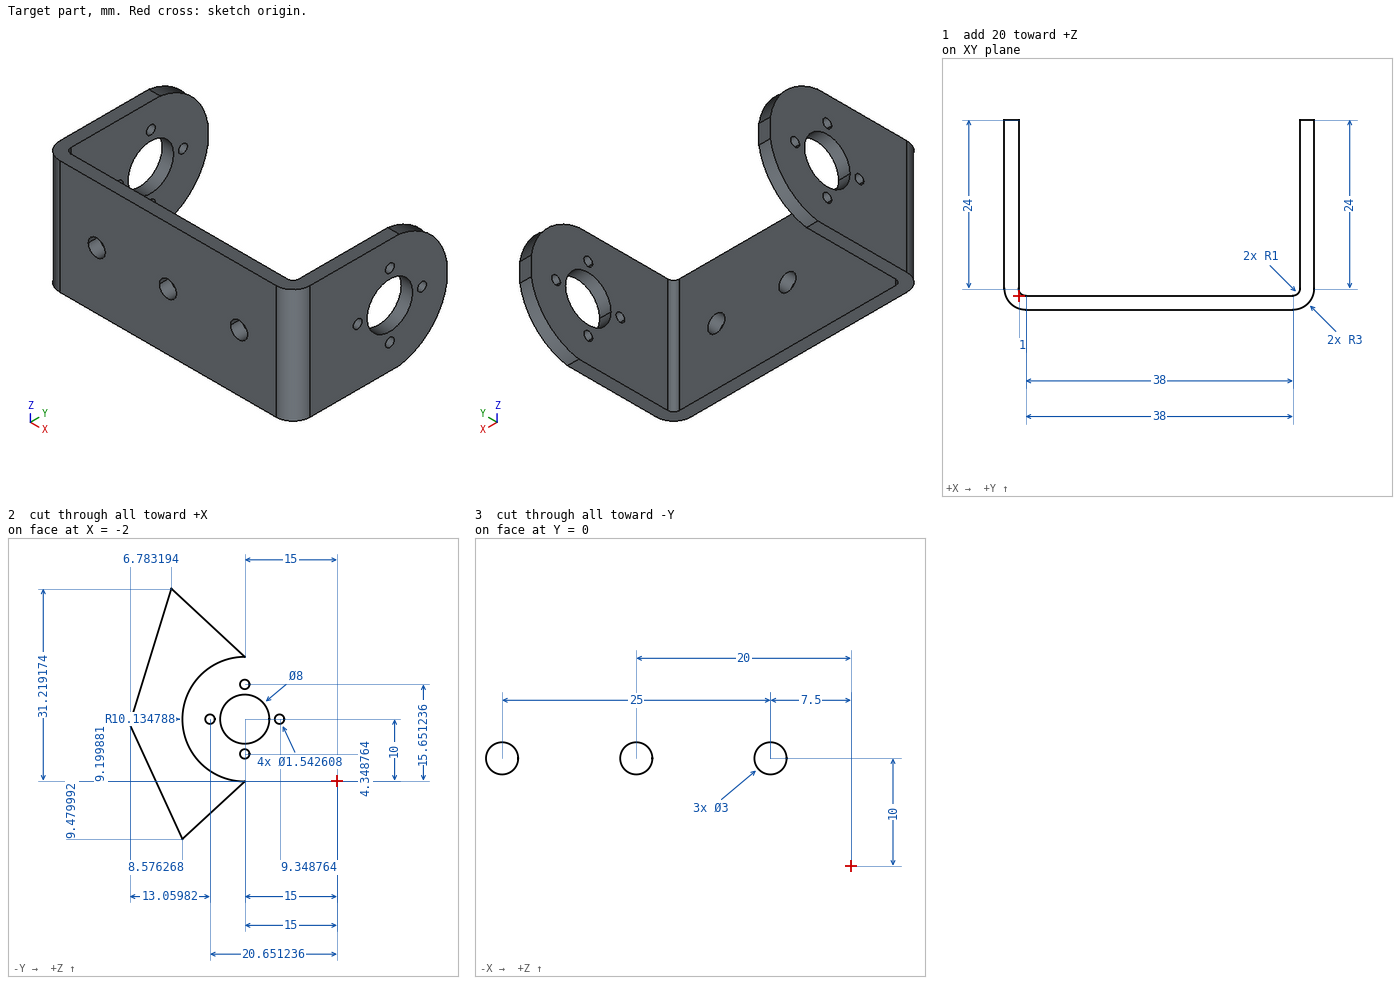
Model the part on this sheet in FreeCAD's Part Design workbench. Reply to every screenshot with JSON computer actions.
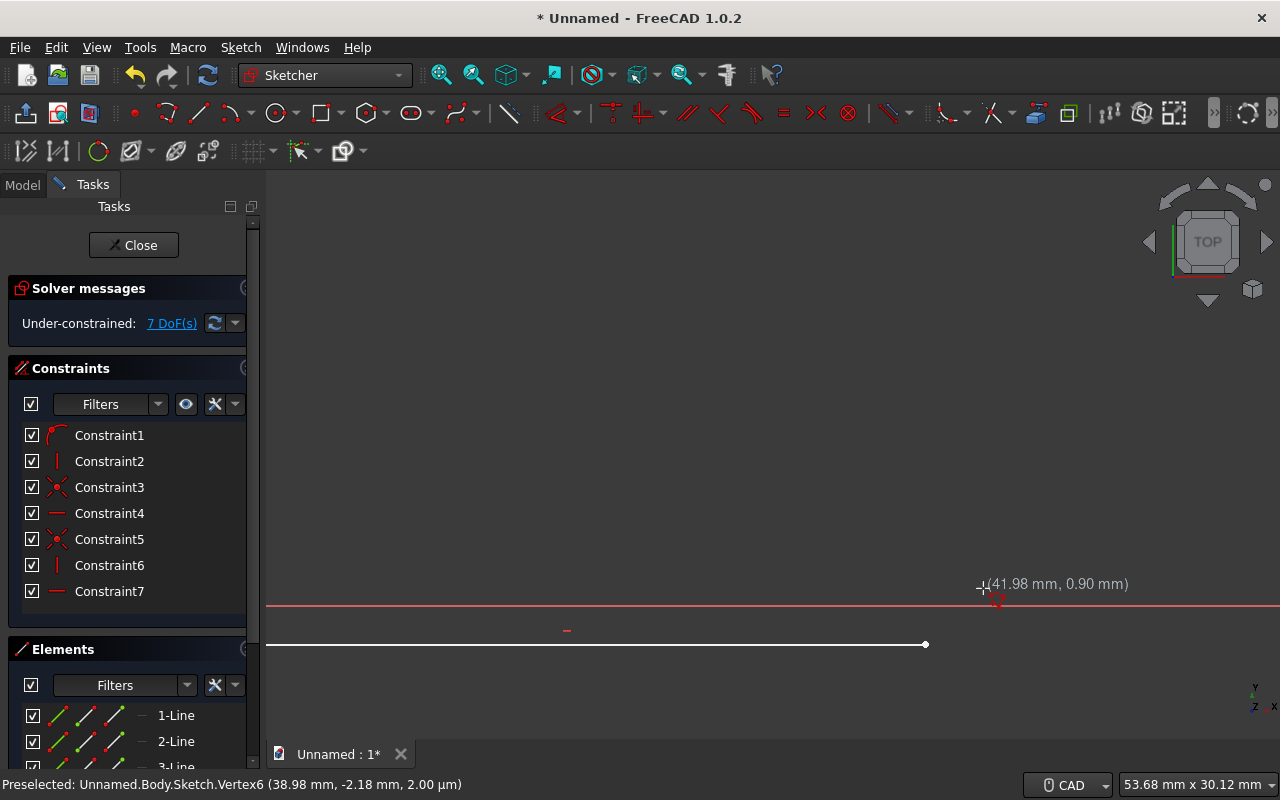
{"action": "left_click", "coordinate": [983, 587]}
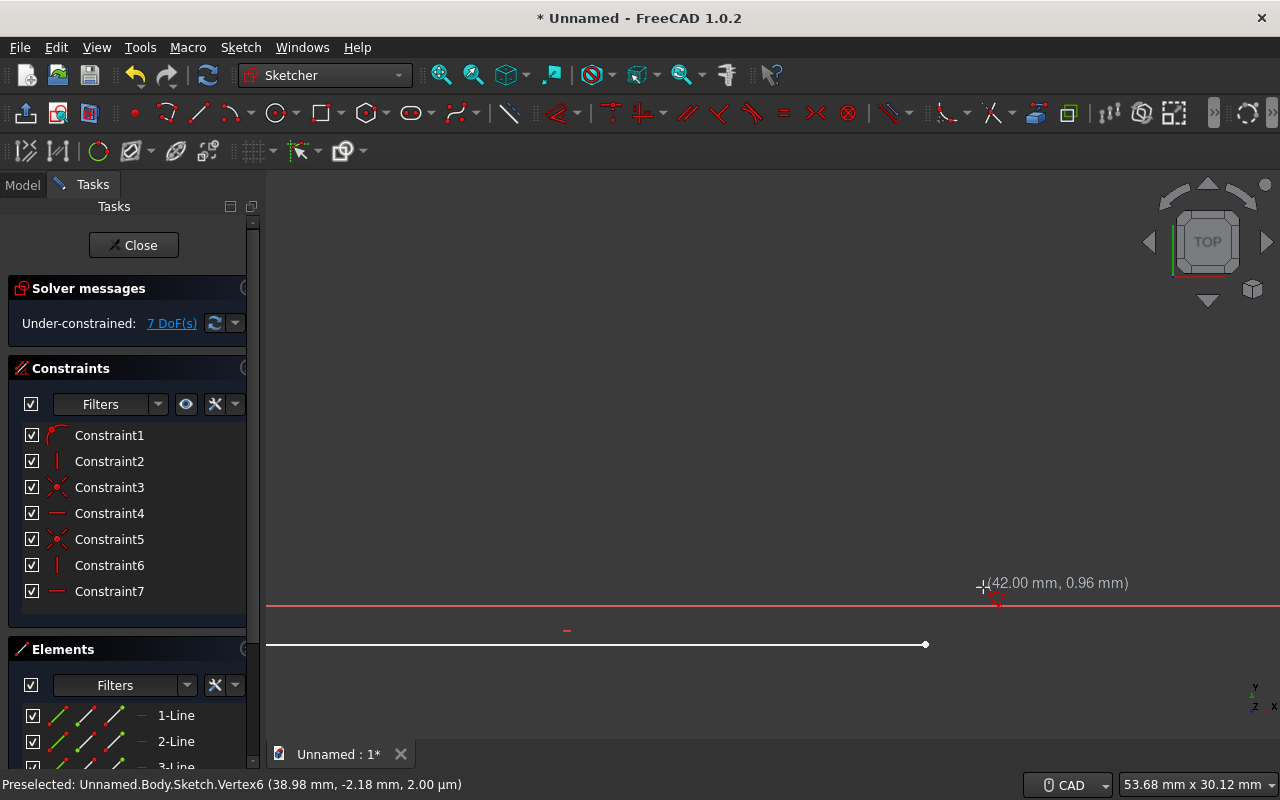
{"action": "scroll", "coordinate": [983, 588], "scroll_direction": "down", "scroll_amount": 2}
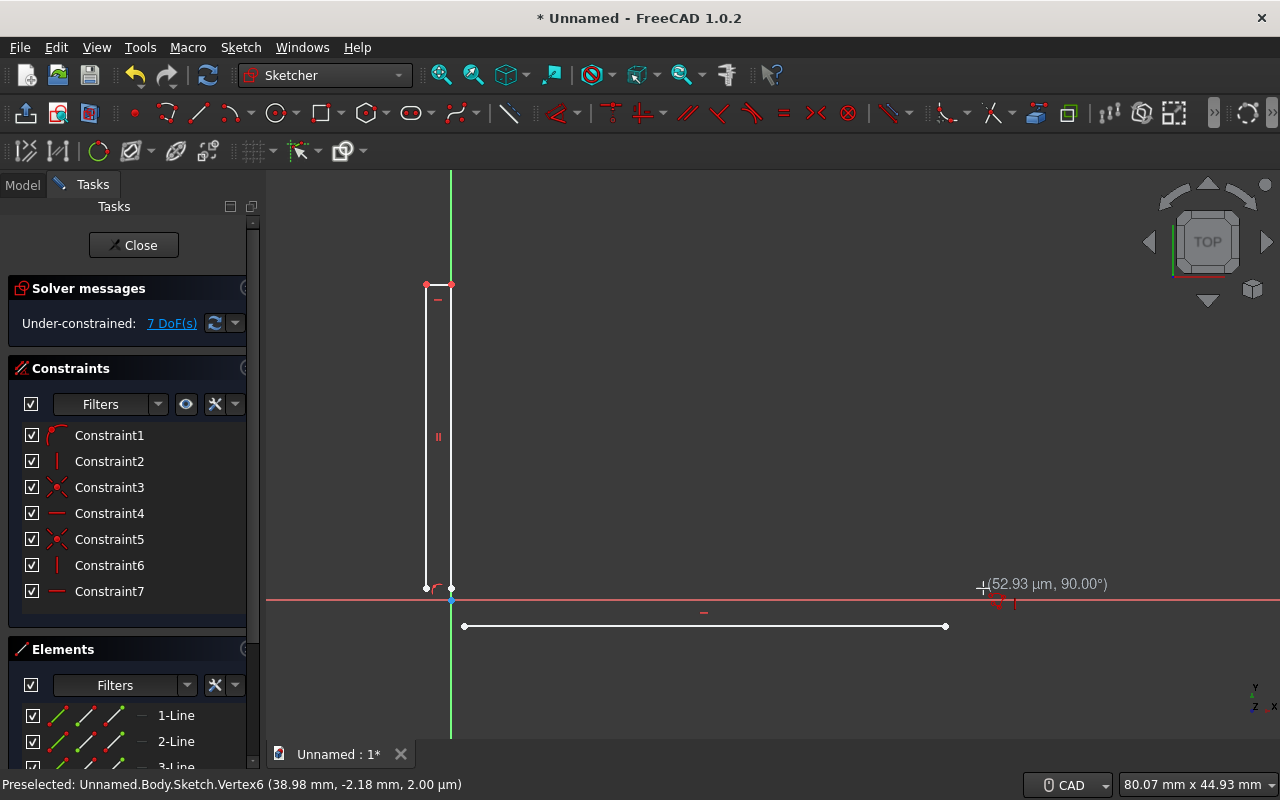
{"action": "left_click", "coordinate": [983, 284]}
{"action": "left_click", "coordinate": [958, 284]}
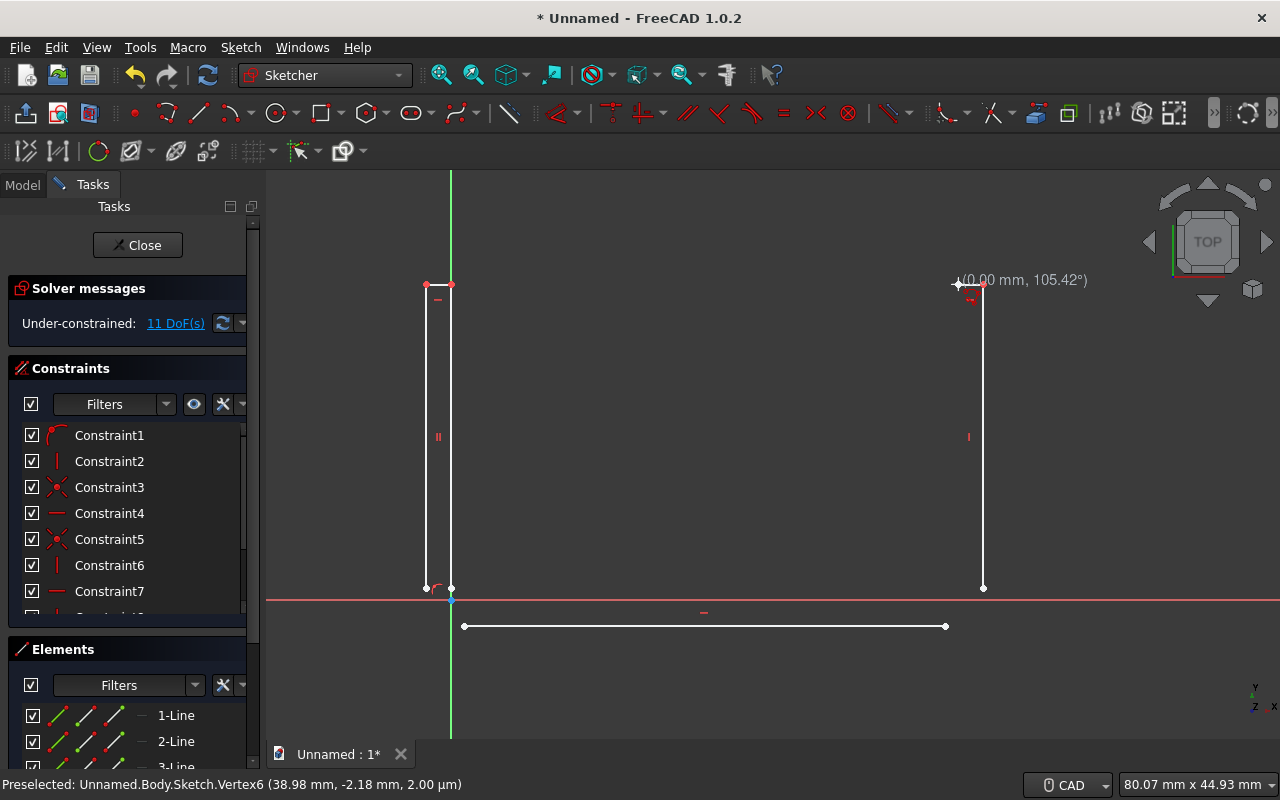
{"action": "scroll", "coordinate": [958, 588], "scroll_direction": "up", "scroll_amount": 2}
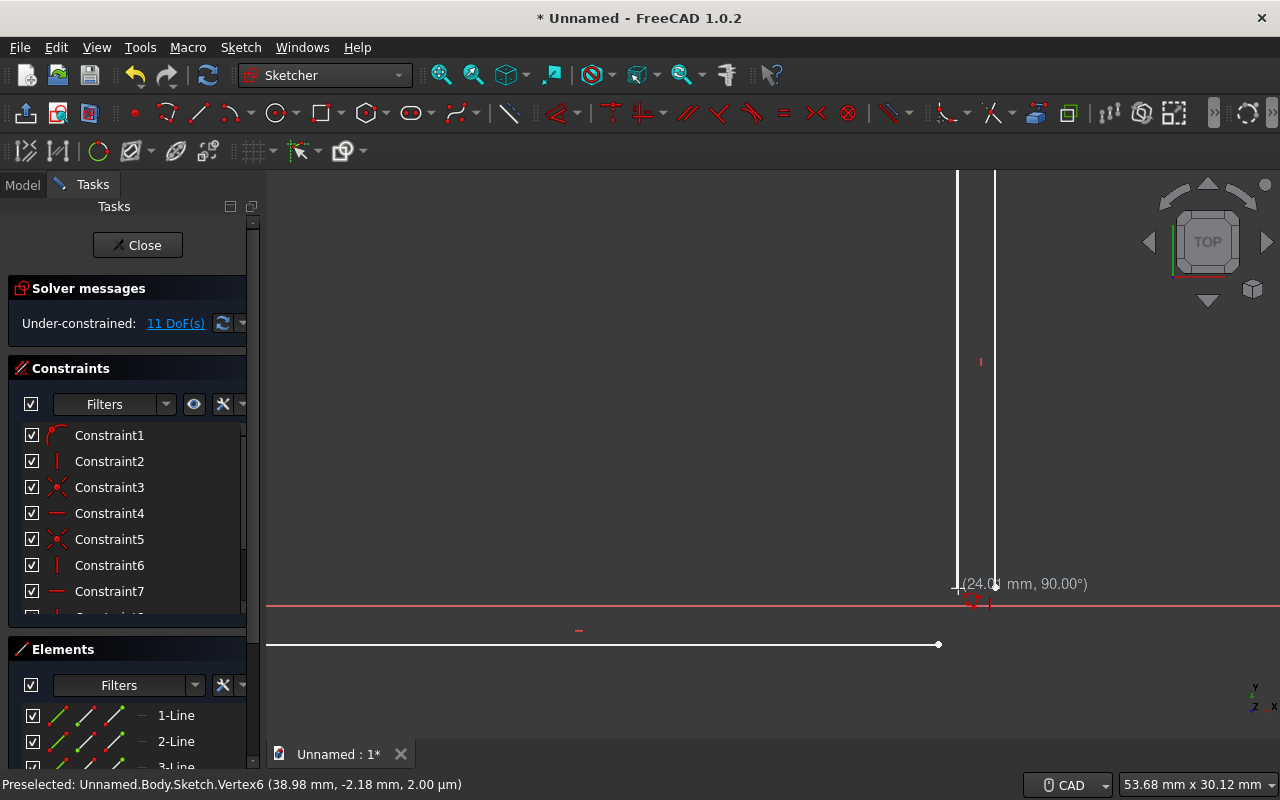
{"action": "left_click", "coordinate": [958, 587]}
{"action": "right_click", "coordinate": [958, 587]}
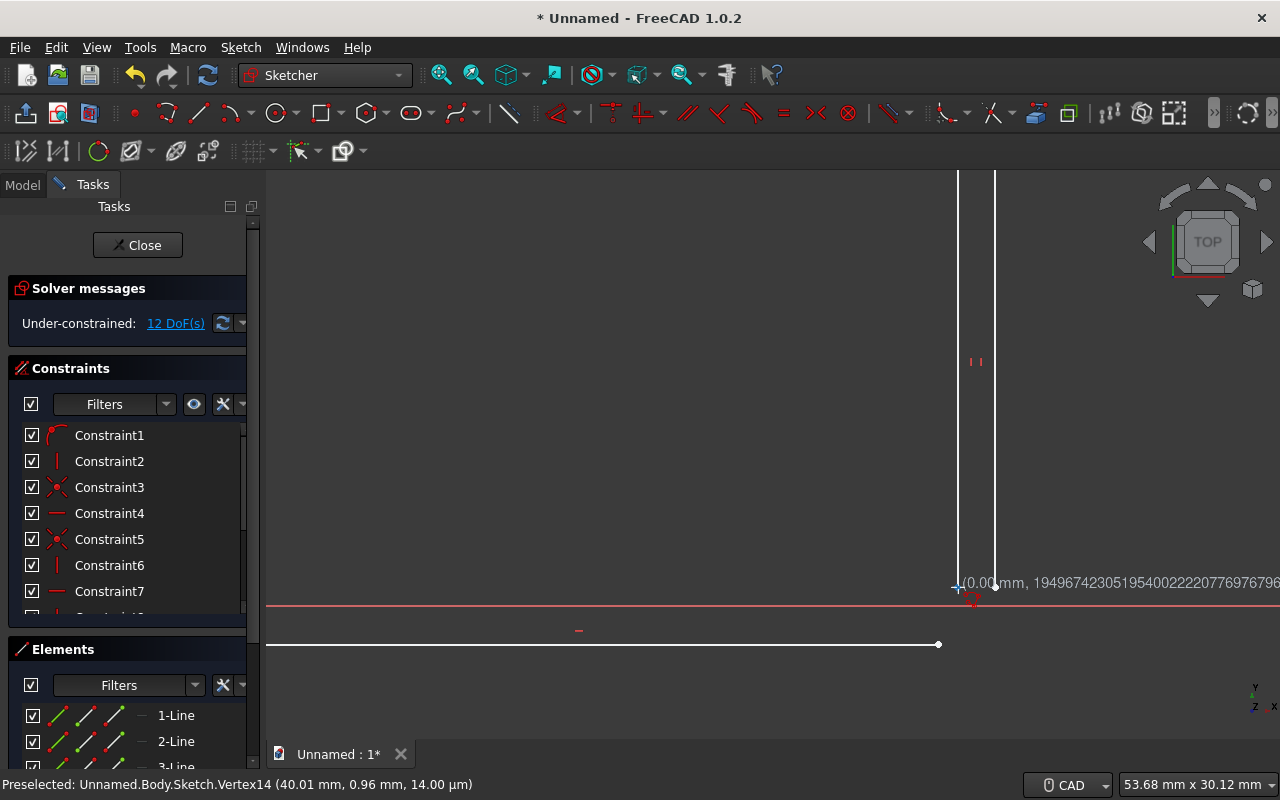
{"action": "left_click", "coordinate": [200, 114]}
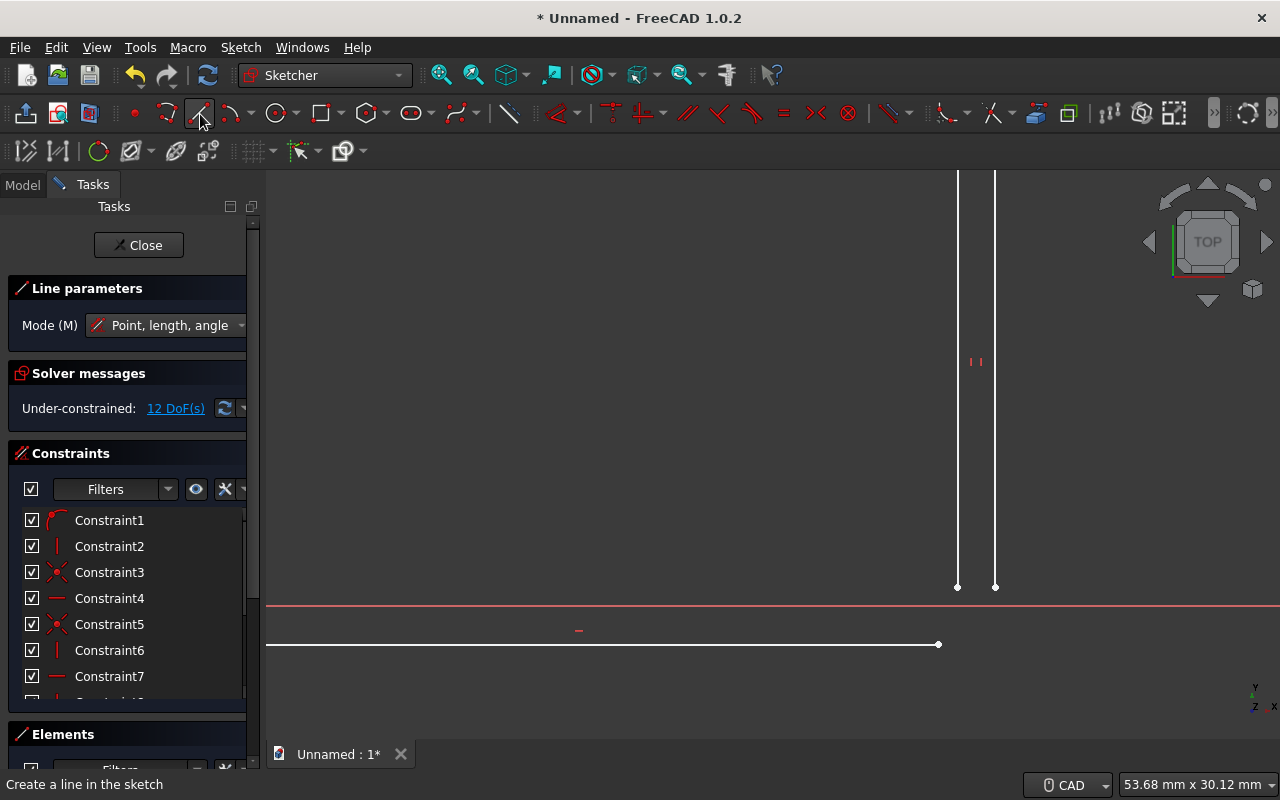
{"action": "left_click", "coordinate": [939, 606]}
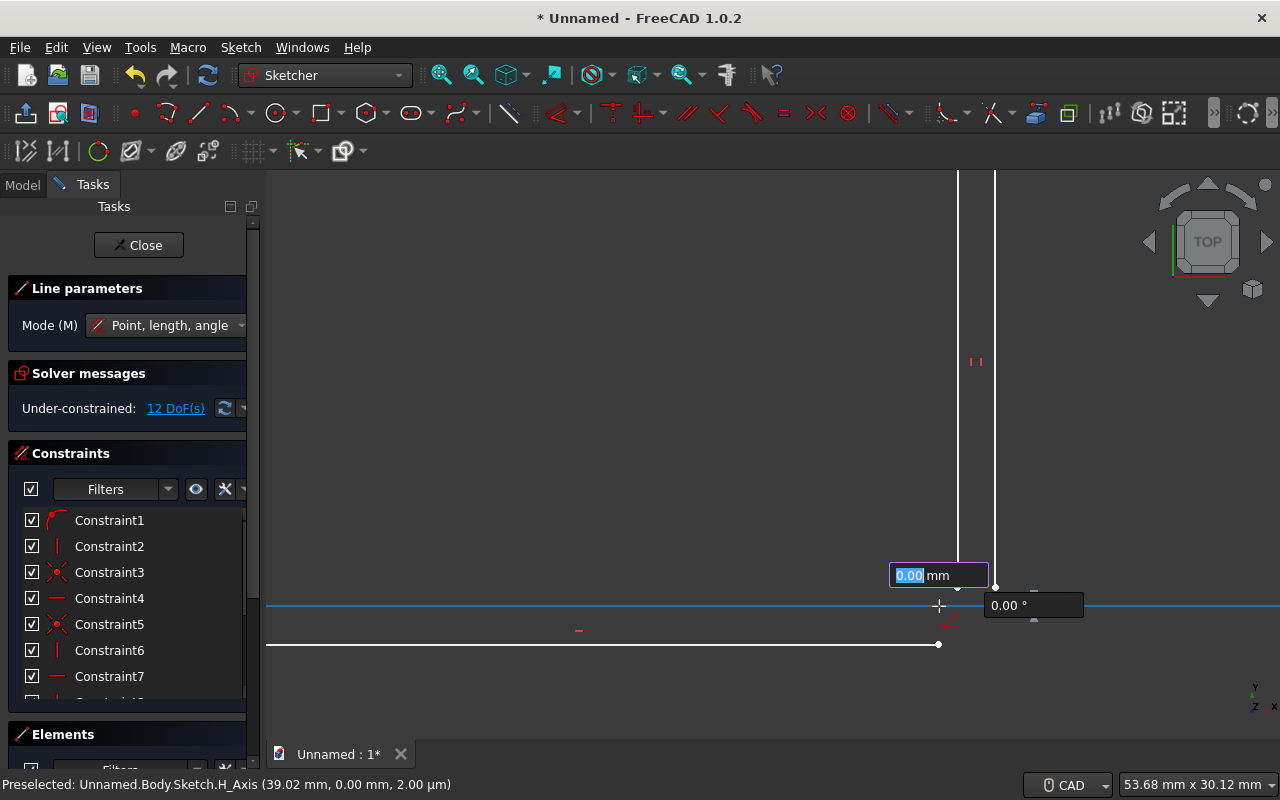
{"action": "scroll", "coordinate": [958, 588], "scroll_direction": "down", "scroll_amount": 2}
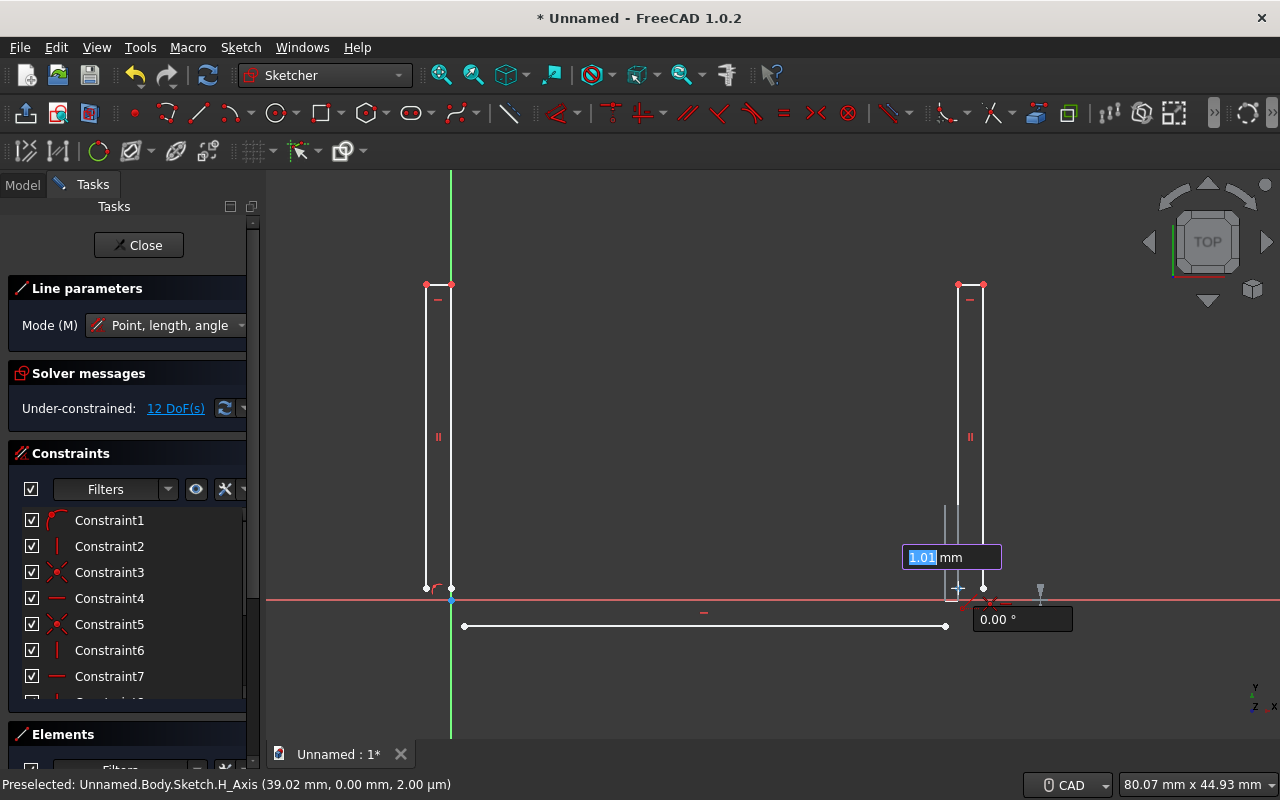
{"action": "scroll", "coordinate": [464, 600], "scroll_direction": "up", "scroll_amount": 2}